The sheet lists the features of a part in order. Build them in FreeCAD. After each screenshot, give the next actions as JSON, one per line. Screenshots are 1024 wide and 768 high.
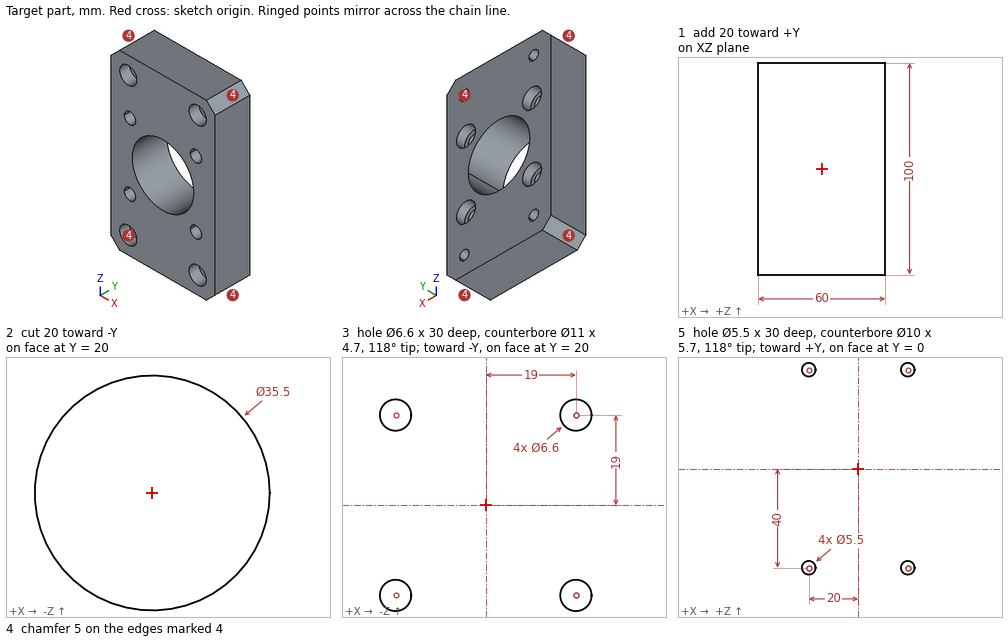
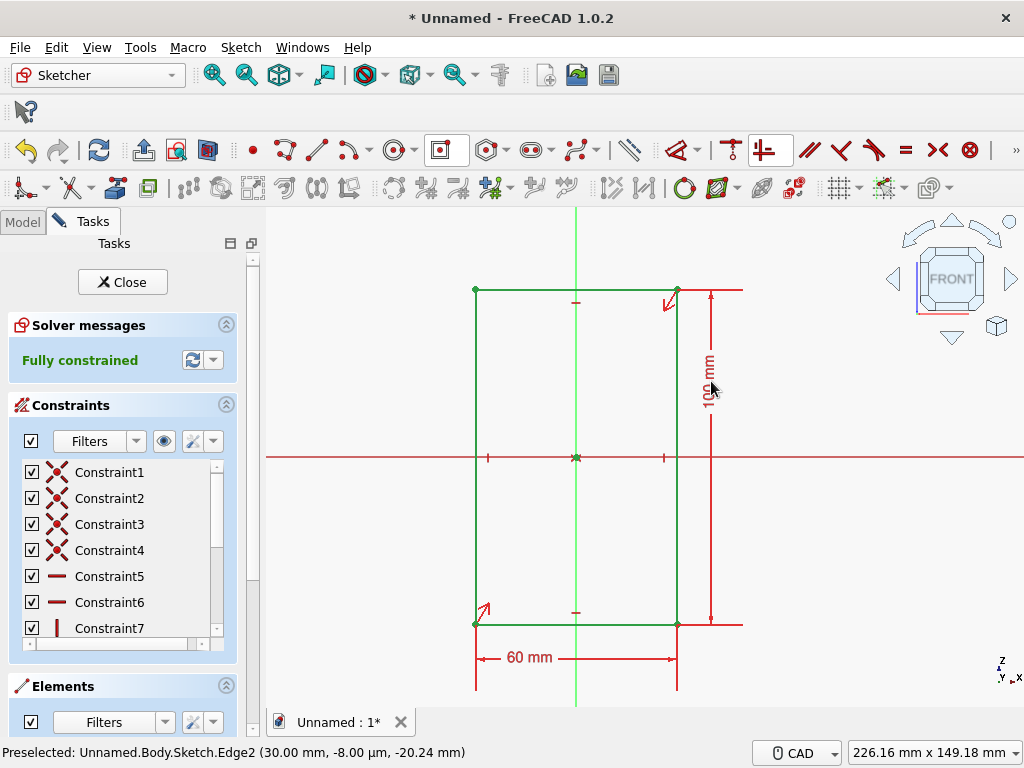
{"action": "left_click", "coordinate": [123, 282]}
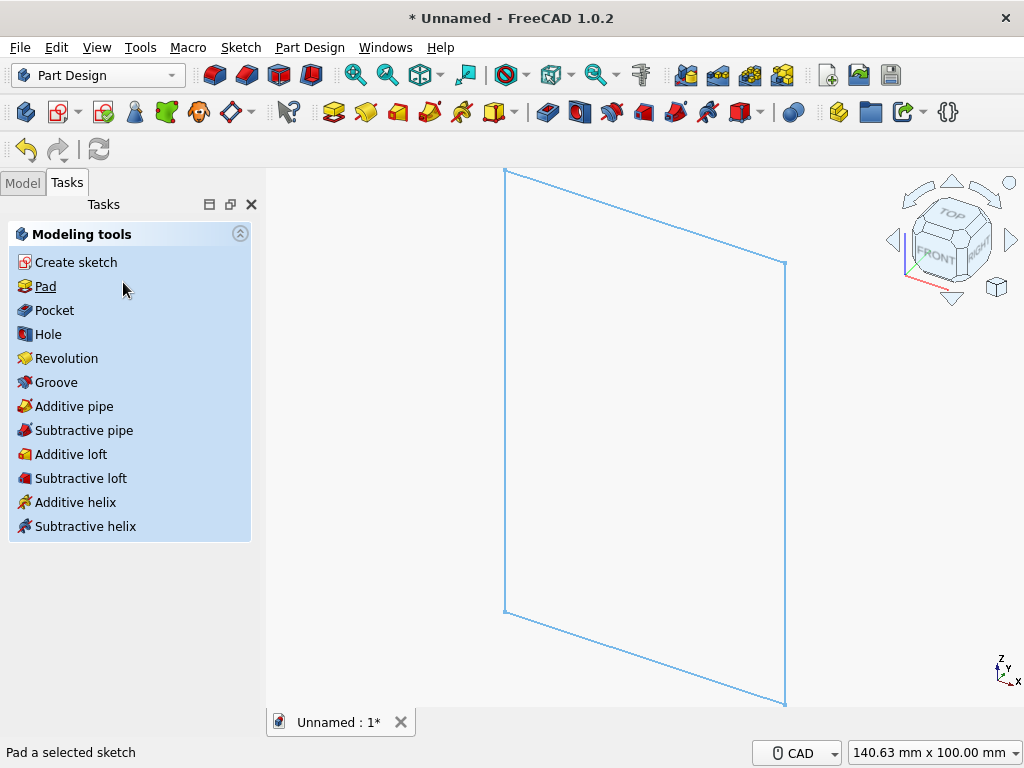
{"action": "left_click", "coordinate": [334, 112]}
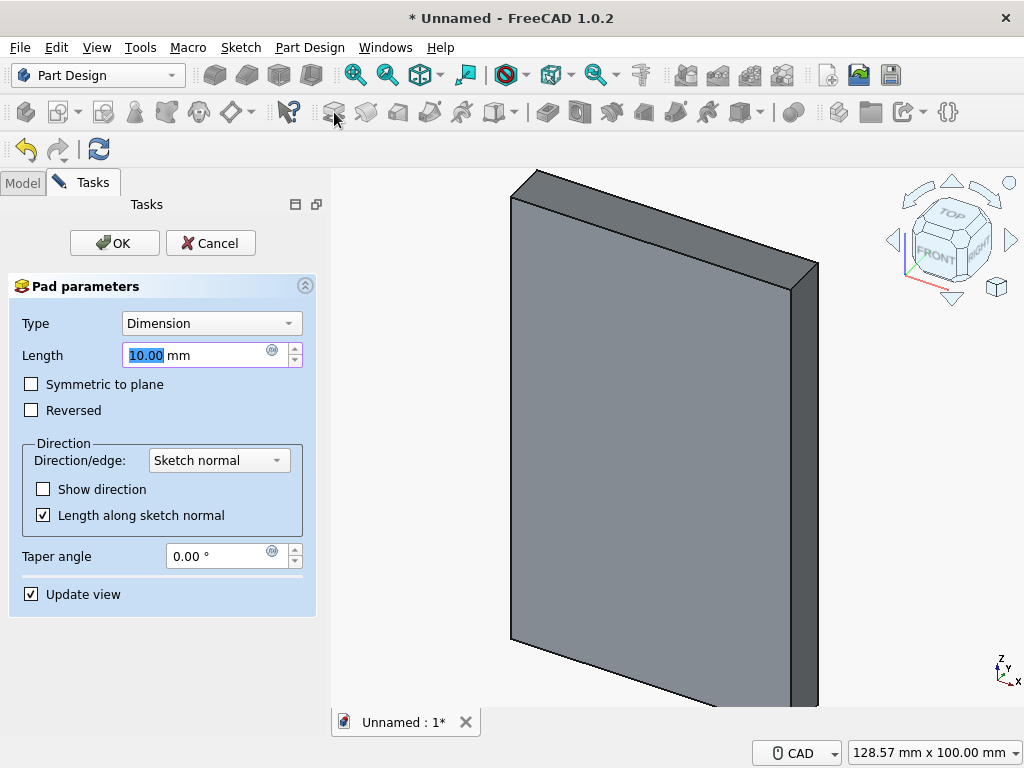
{"action": "type", "text": "20"}
{"action": "key", "text": "Tab"}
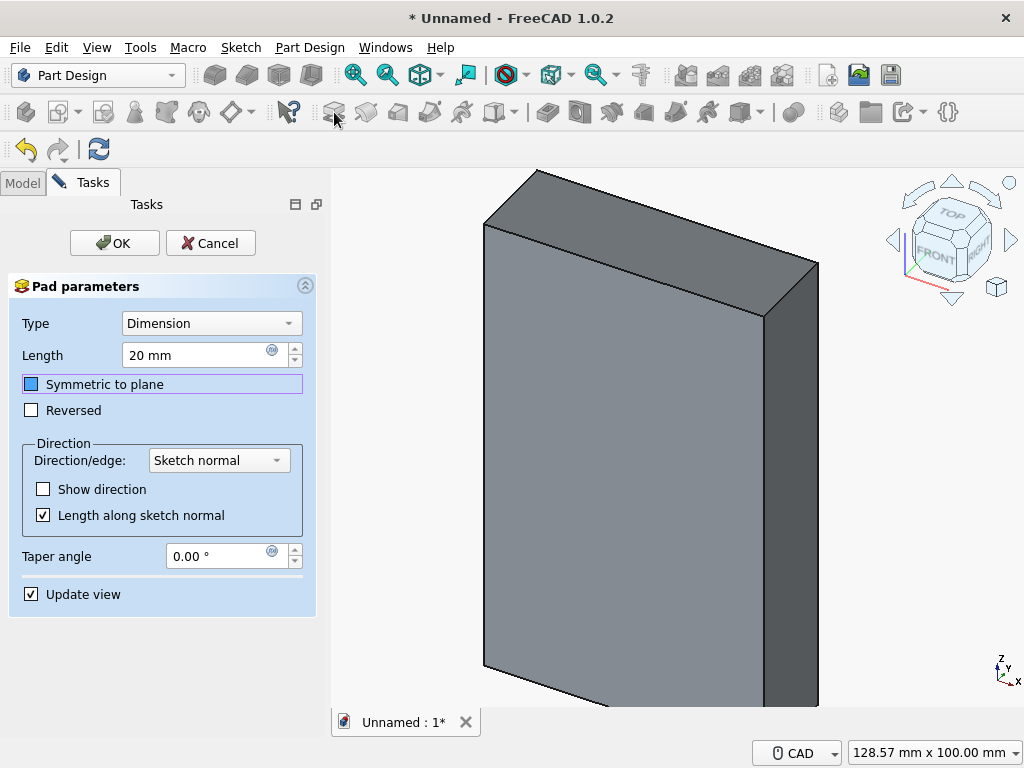
{"action": "left_click", "coordinate": [30, 410]}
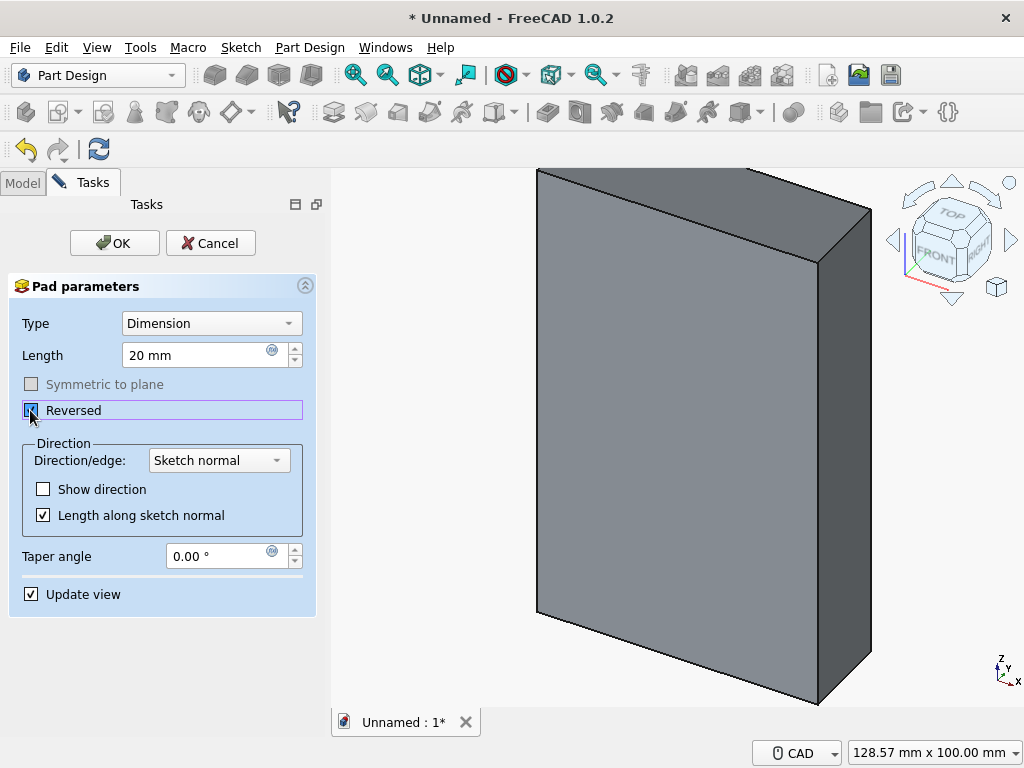
{"action": "left_click", "coordinate": [115, 243]}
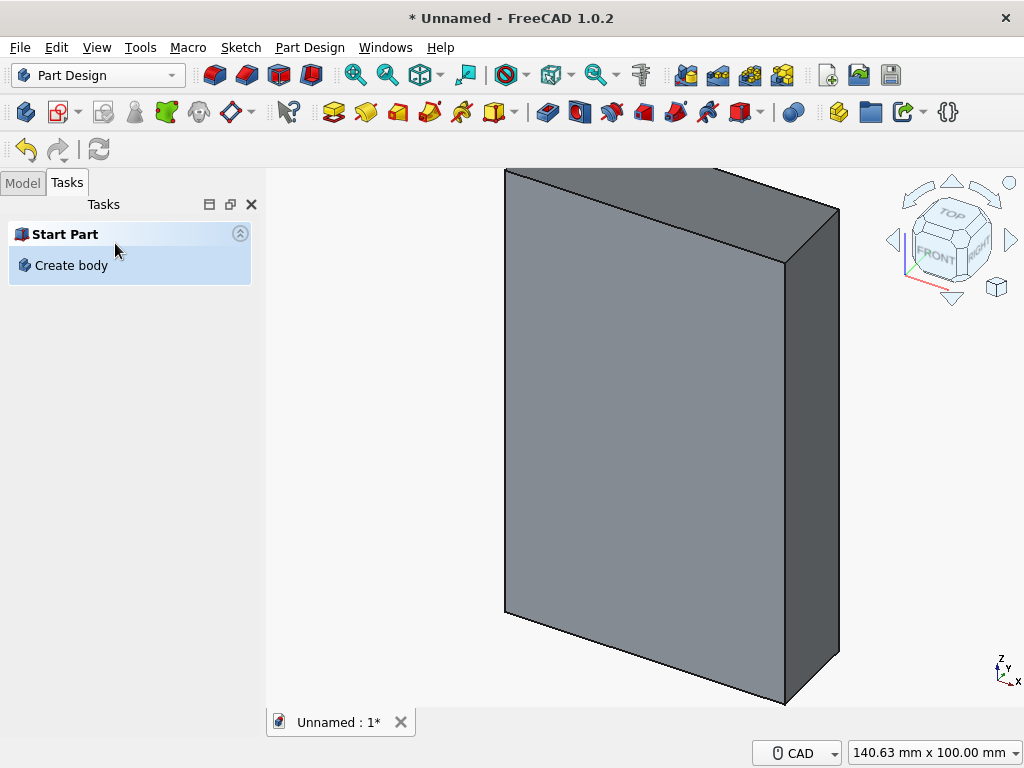
{"action": "key", "text": "v f"}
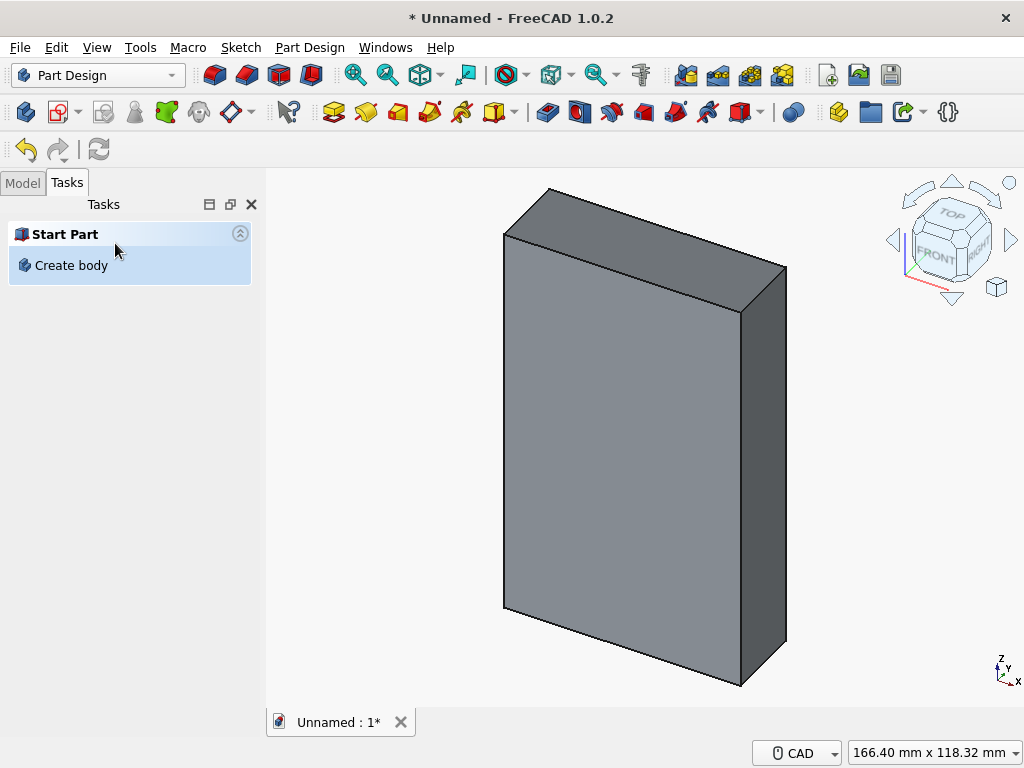
{"action": "key", "text": "4"}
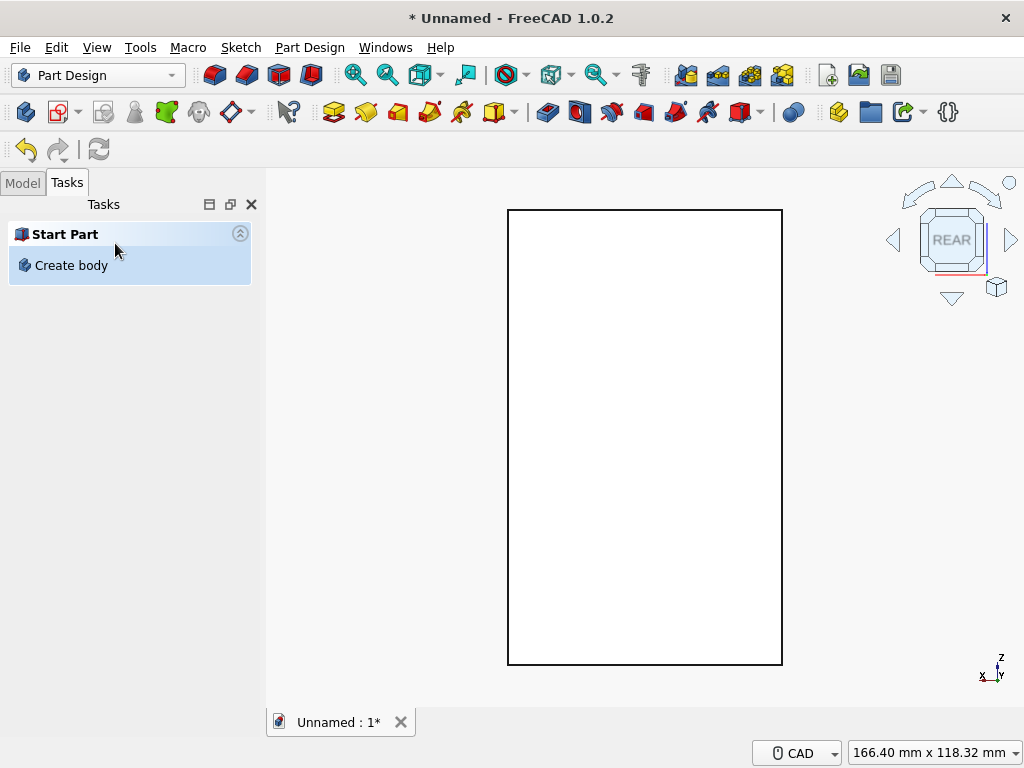
{"action": "left_click", "coordinate": [645, 371]}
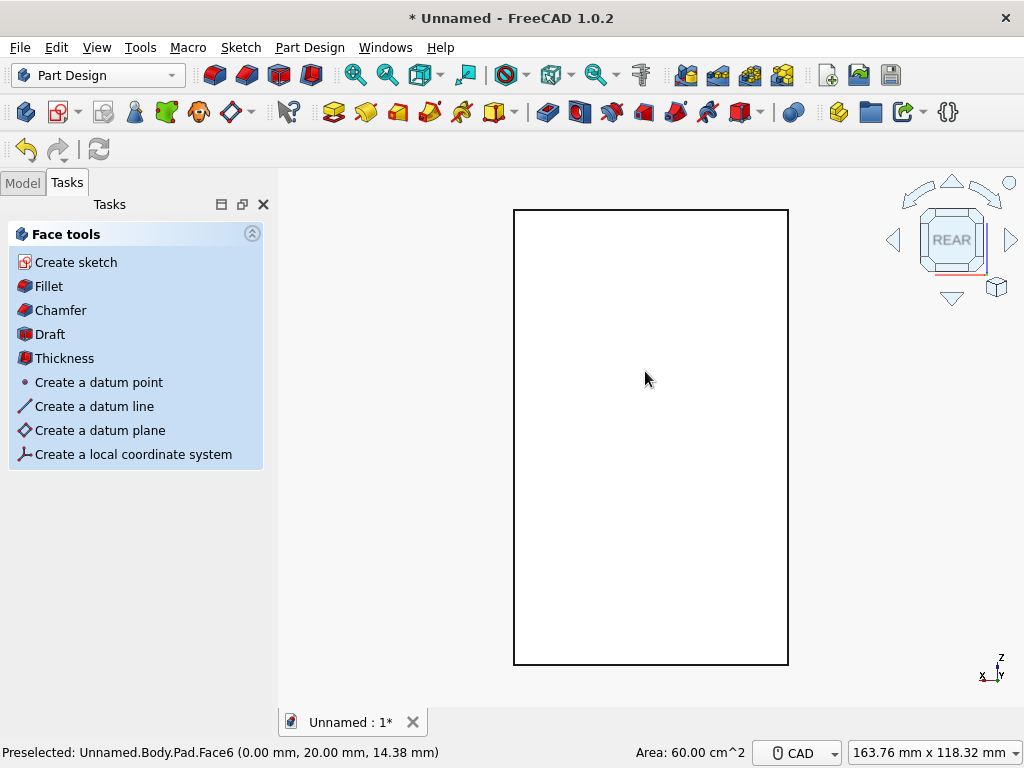
{"action": "left_click", "coordinate": [58, 112]}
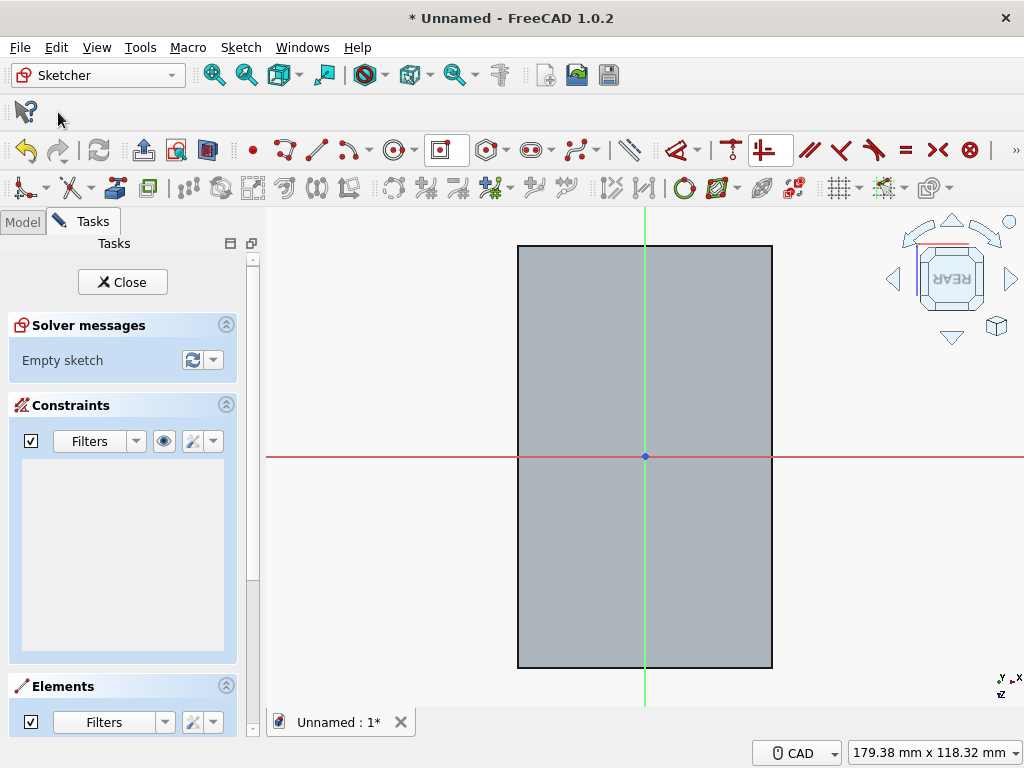
{"action": "scroll", "coordinate": [701, 457], "scroll_direction": "up", "scroll_amount": 4}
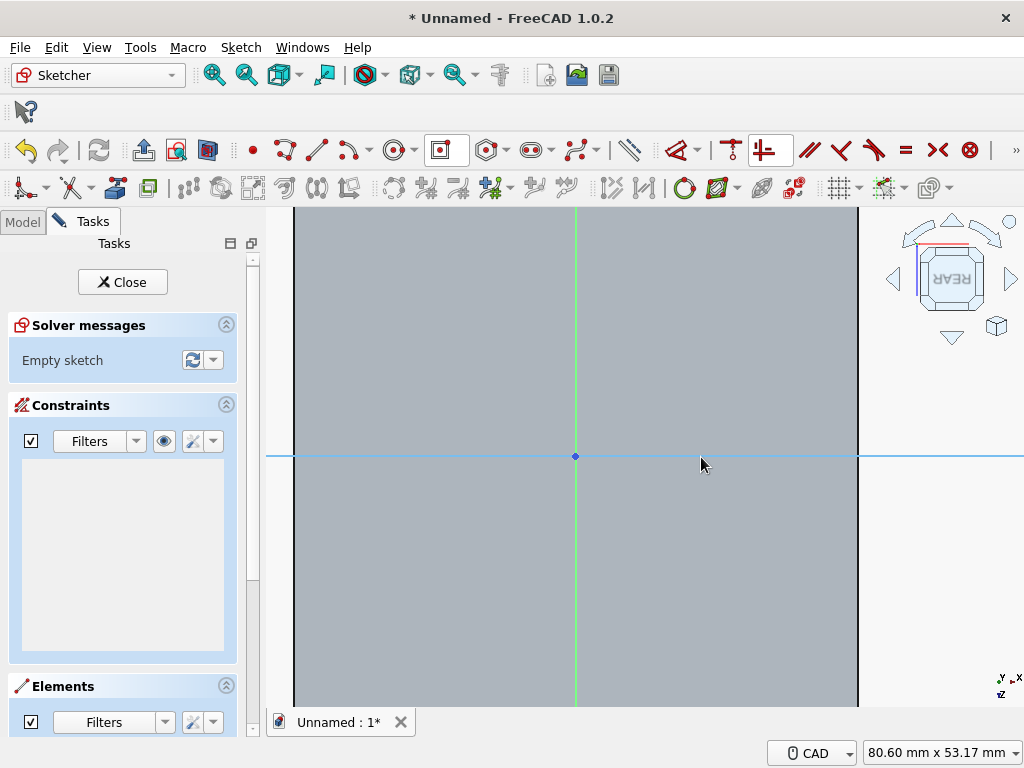
{"action": "left_click", "coordinate": [394, 150]}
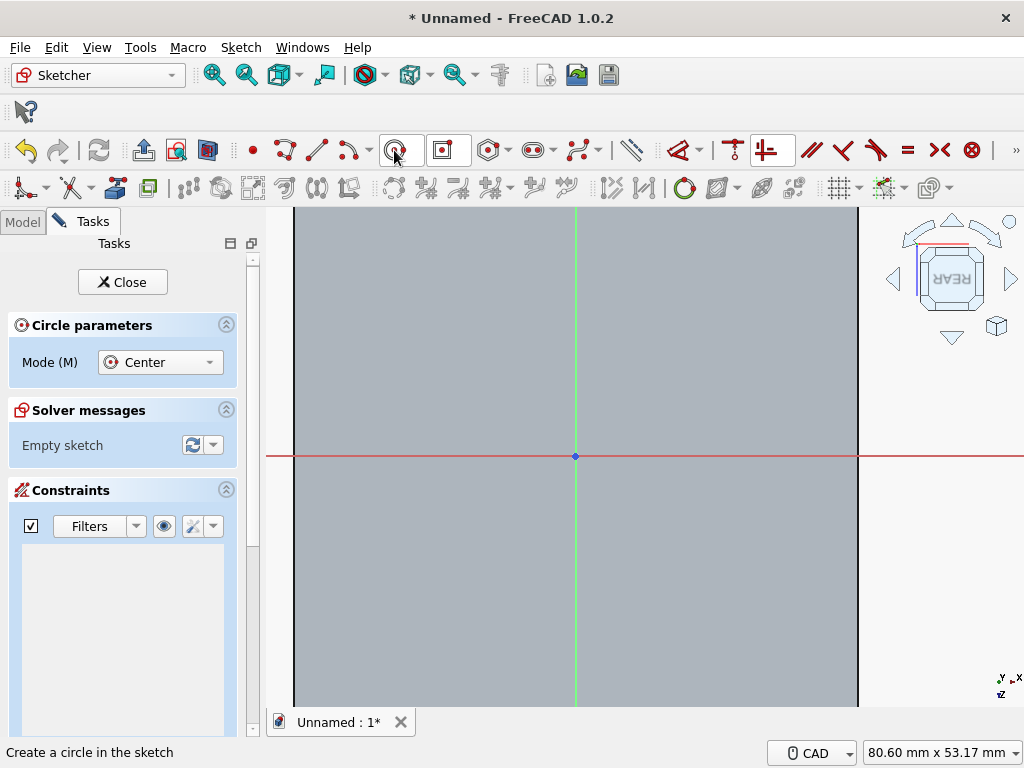
{"action": "left_click", "coordinate": [576, 456]}
{"action": "left_click", "coordinate": [694, 338]}
{"action": "key", "text": "Escape"}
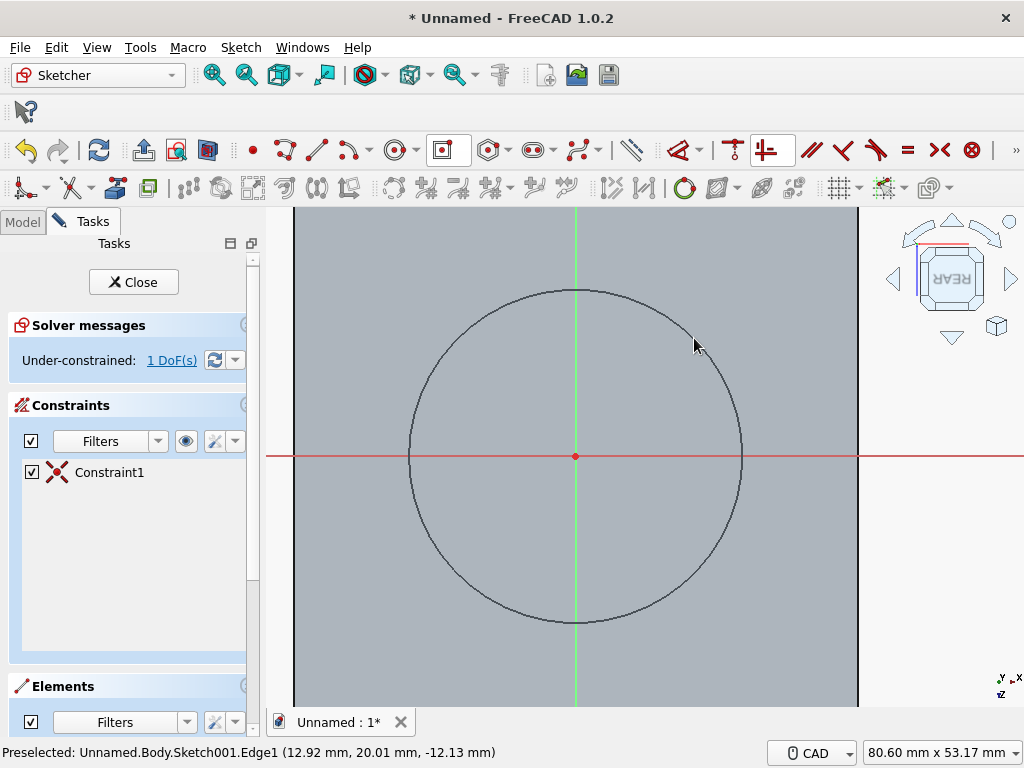
{"action": "left_click", "coordinate": [678, 150]}